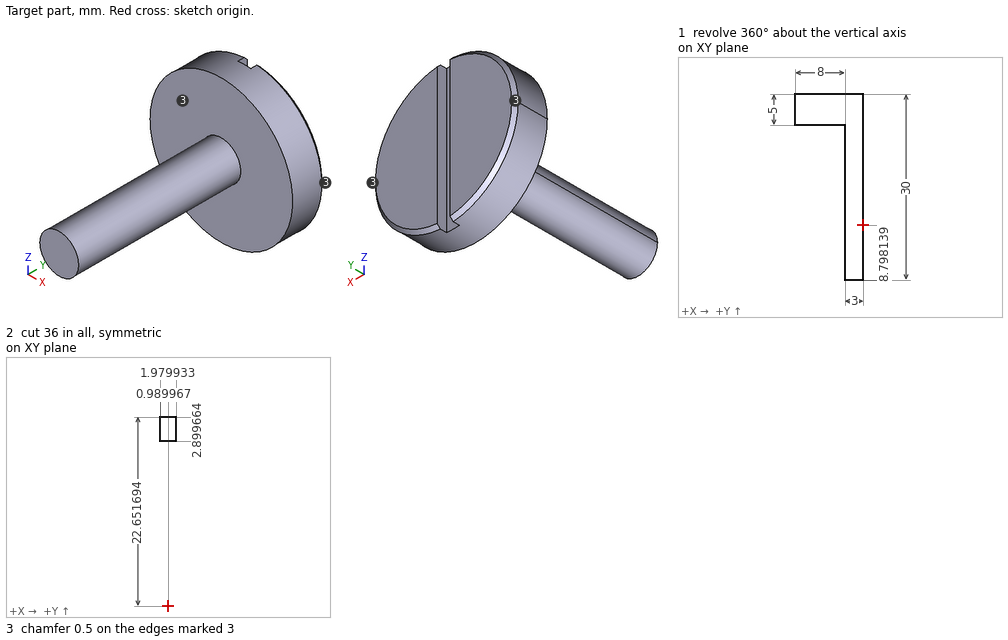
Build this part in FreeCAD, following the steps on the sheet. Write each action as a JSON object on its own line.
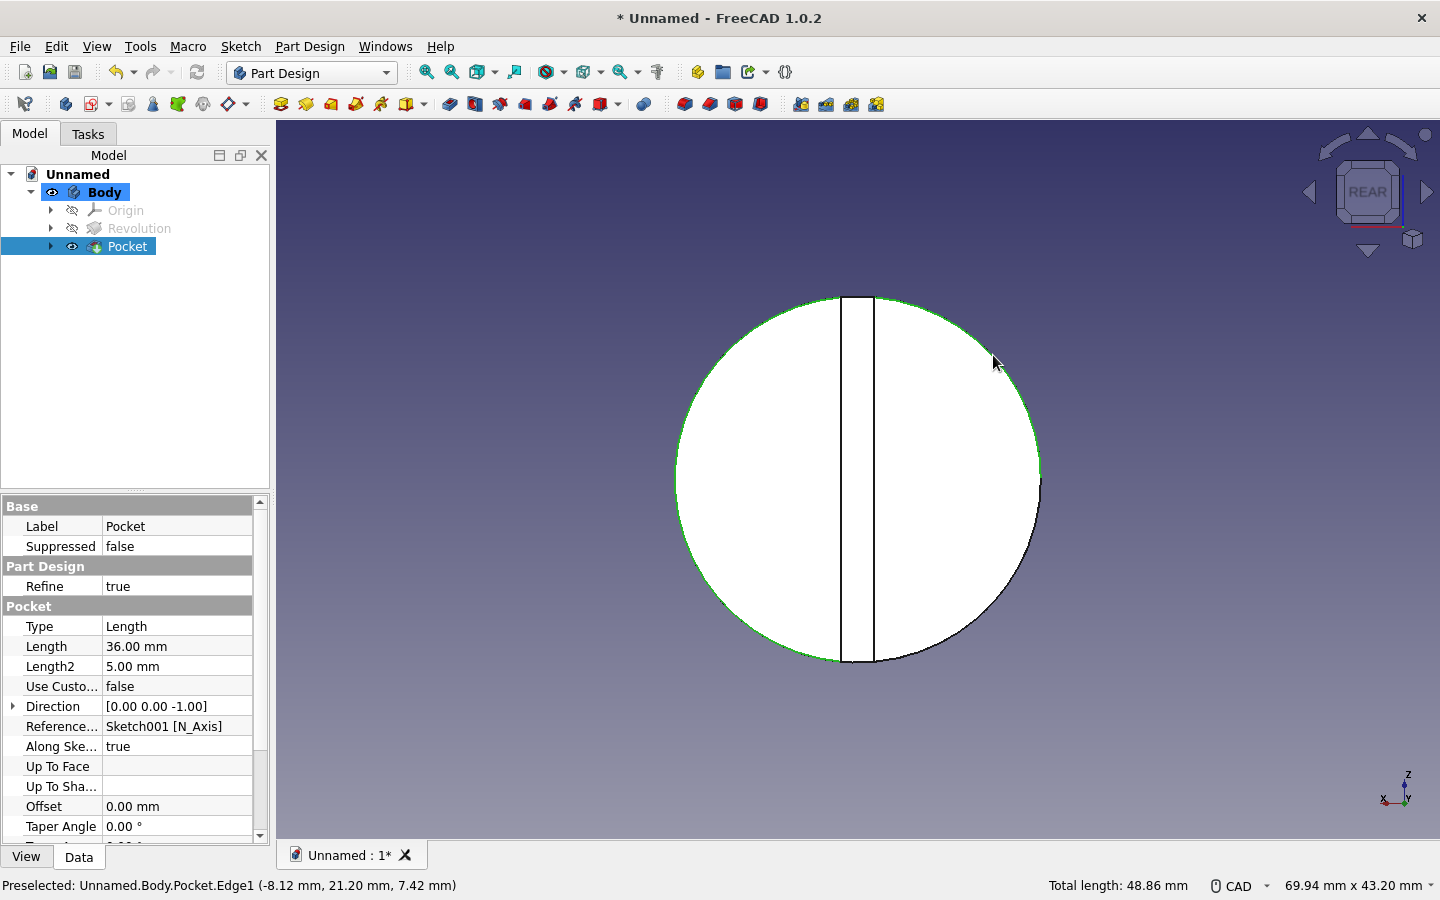
{"action": "left_click", "coordinate": [710, 104]}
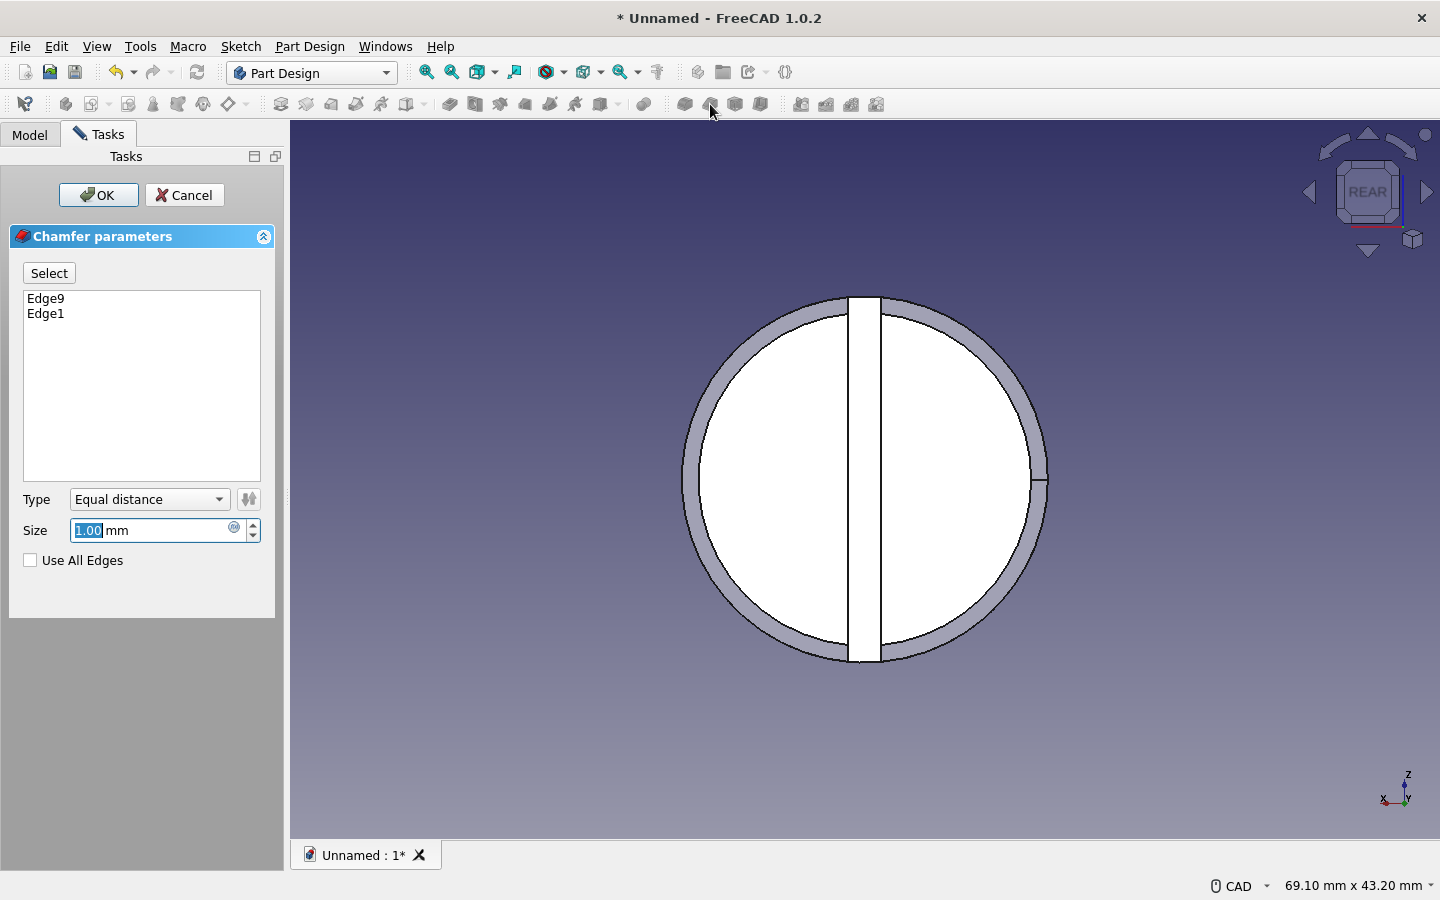
{"action": "type", "text": "0.5"}
{"action": "key", "text": "Tab"}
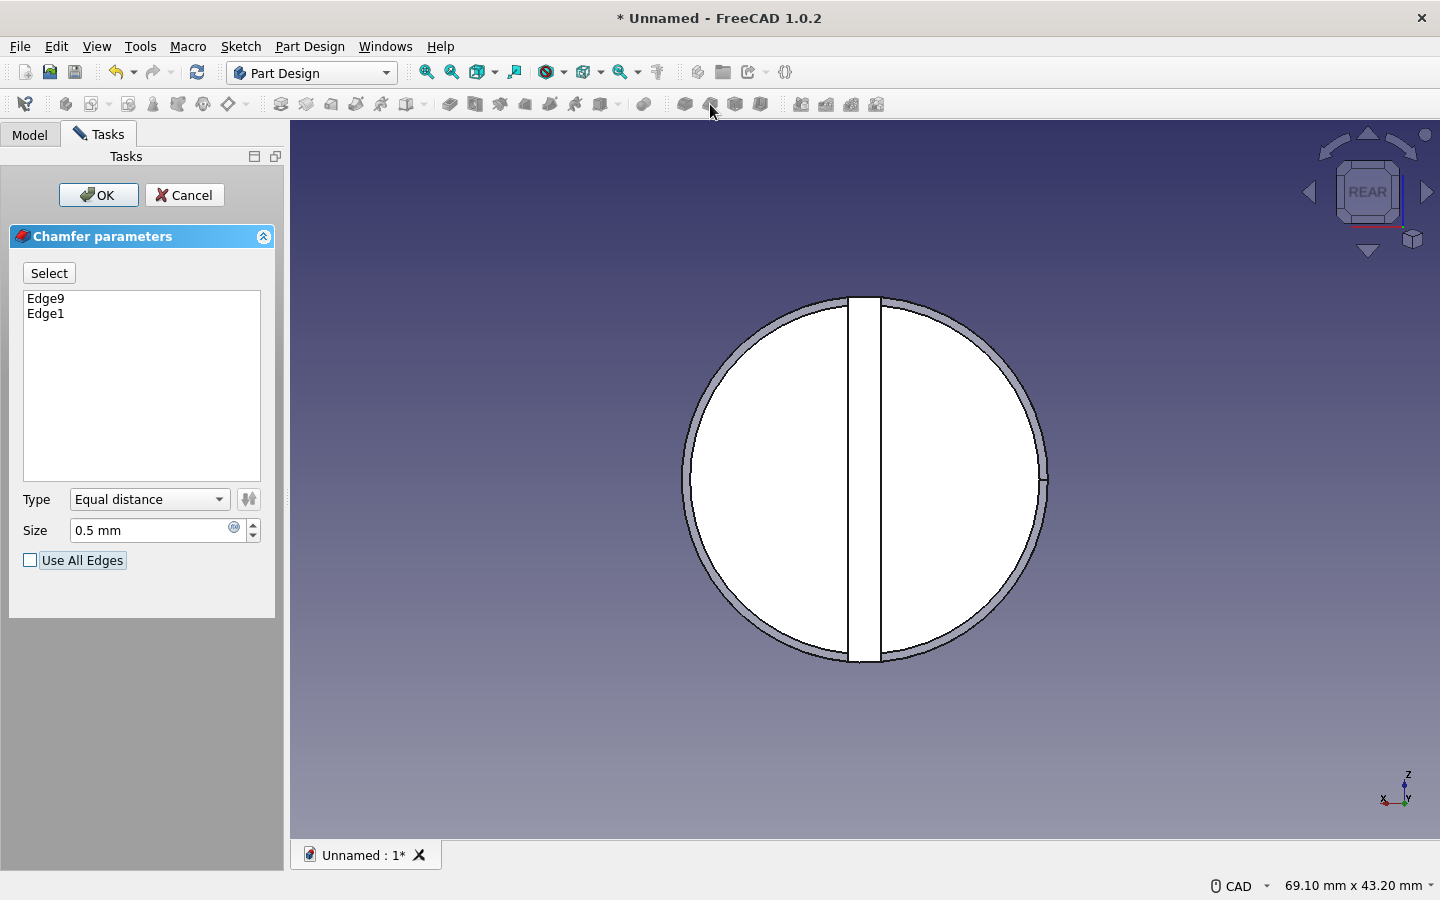
{"action": "left_click", "coordinate": [99, 195]}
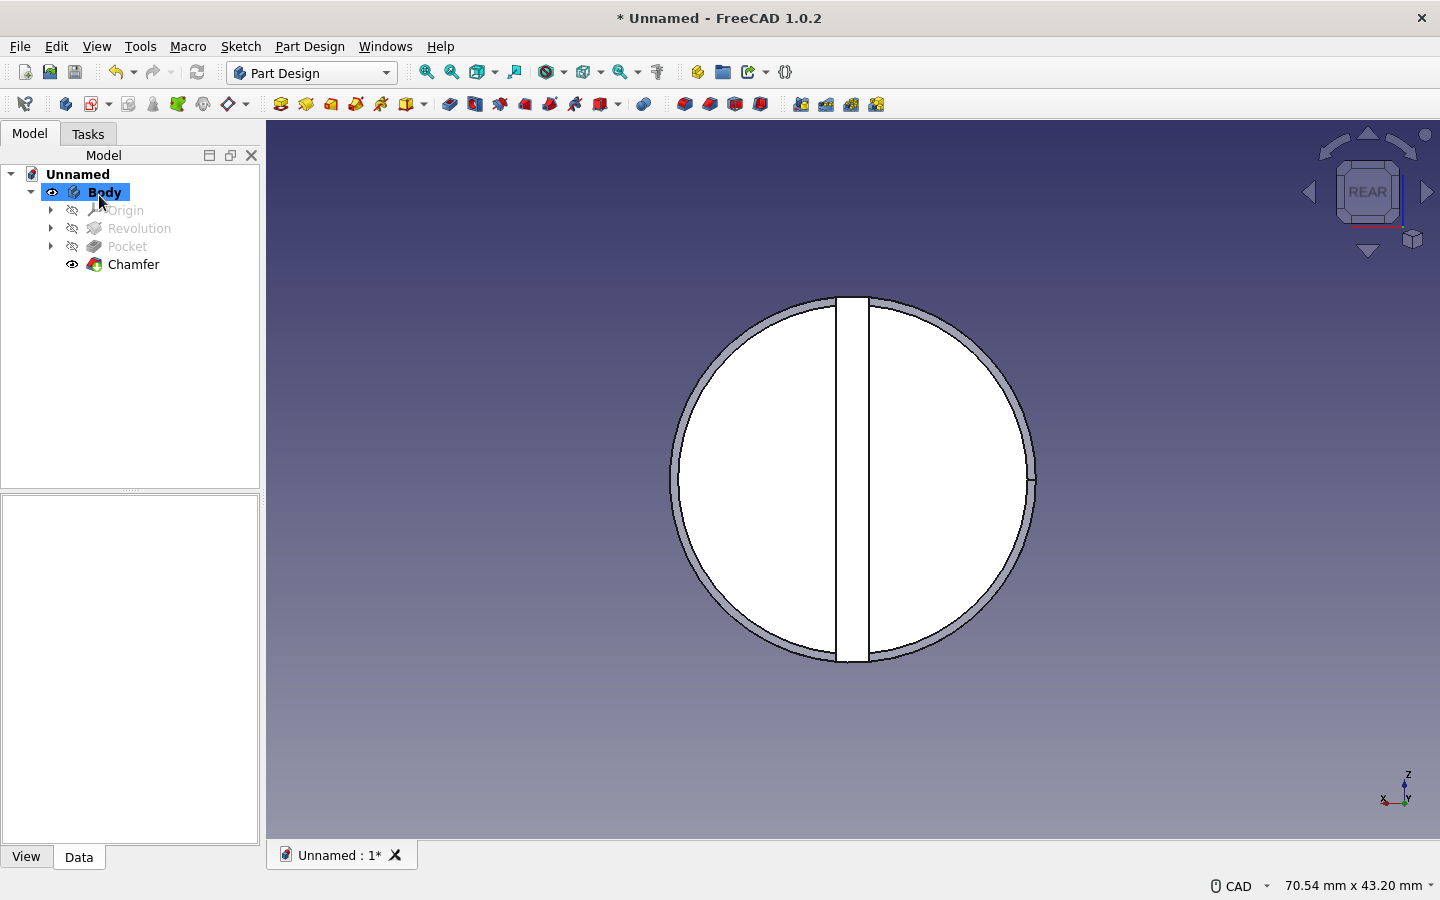
{"action": "key", "text": "0"}